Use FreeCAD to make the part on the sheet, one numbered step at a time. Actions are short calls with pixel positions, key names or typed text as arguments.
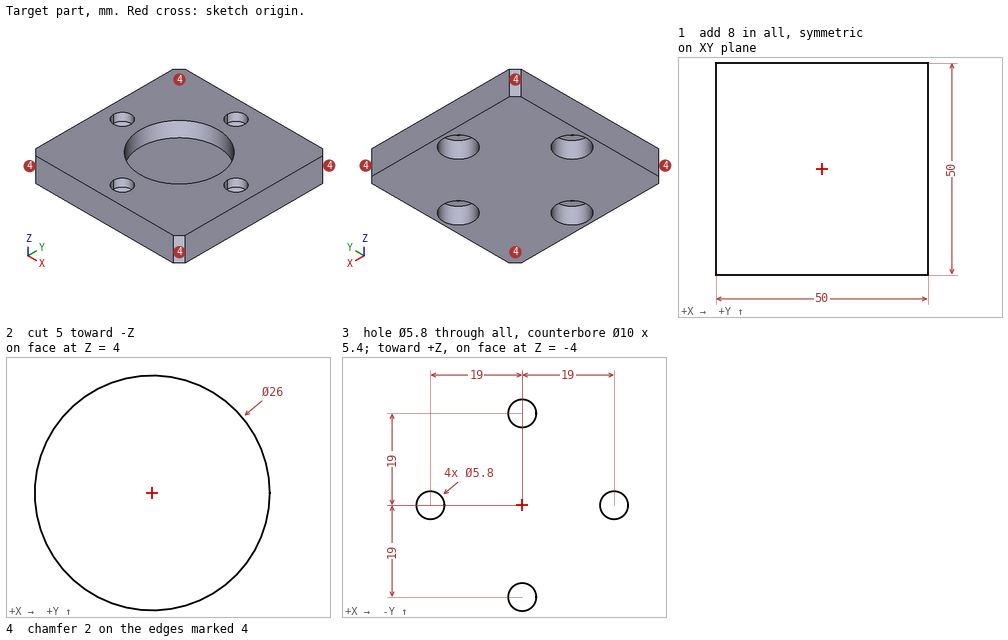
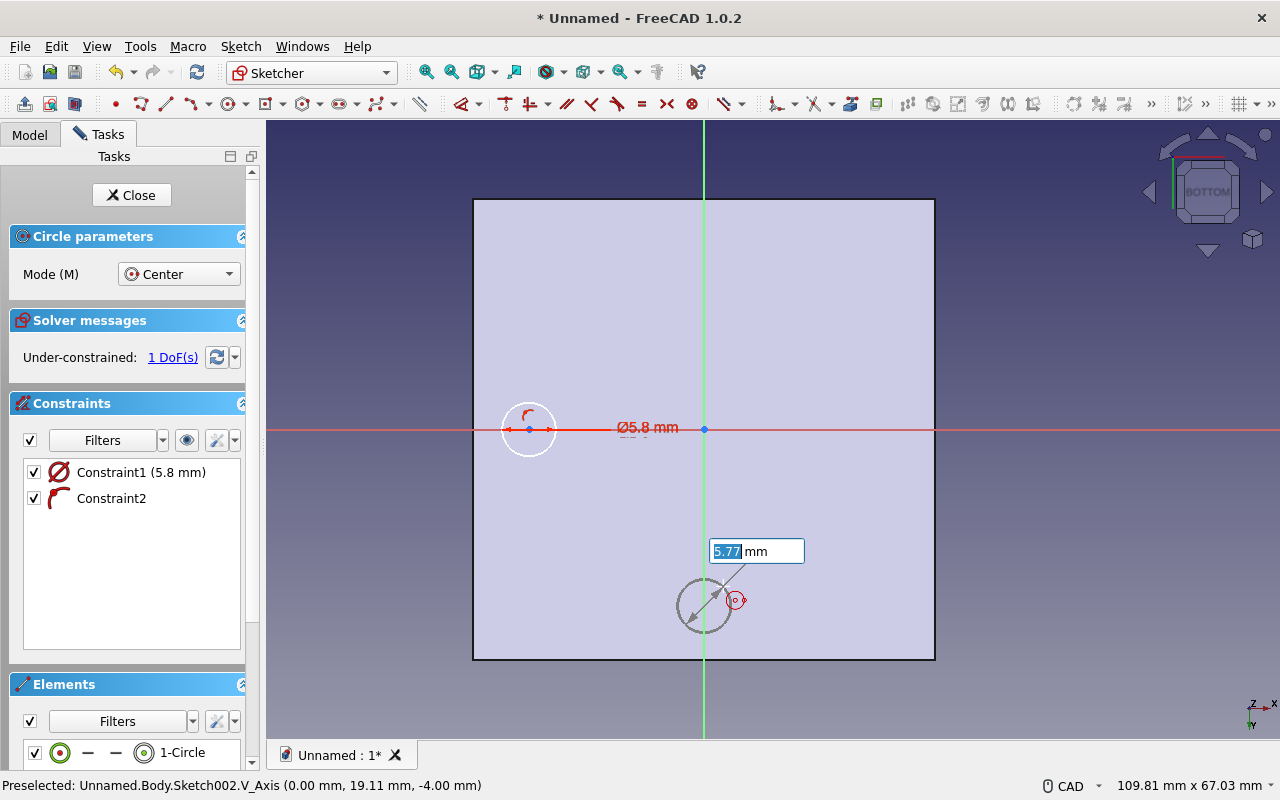
text(5.8)
key(Return)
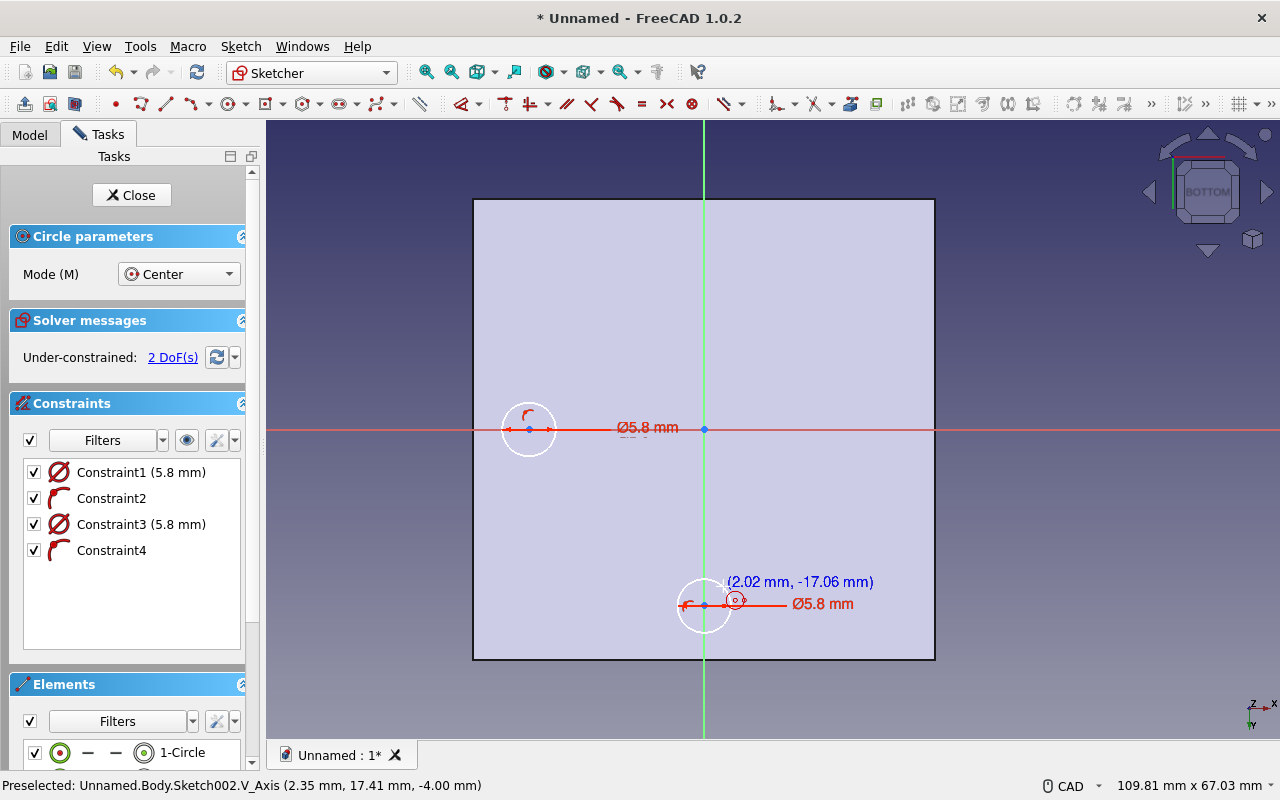
click(880, 430)
move(899, 411)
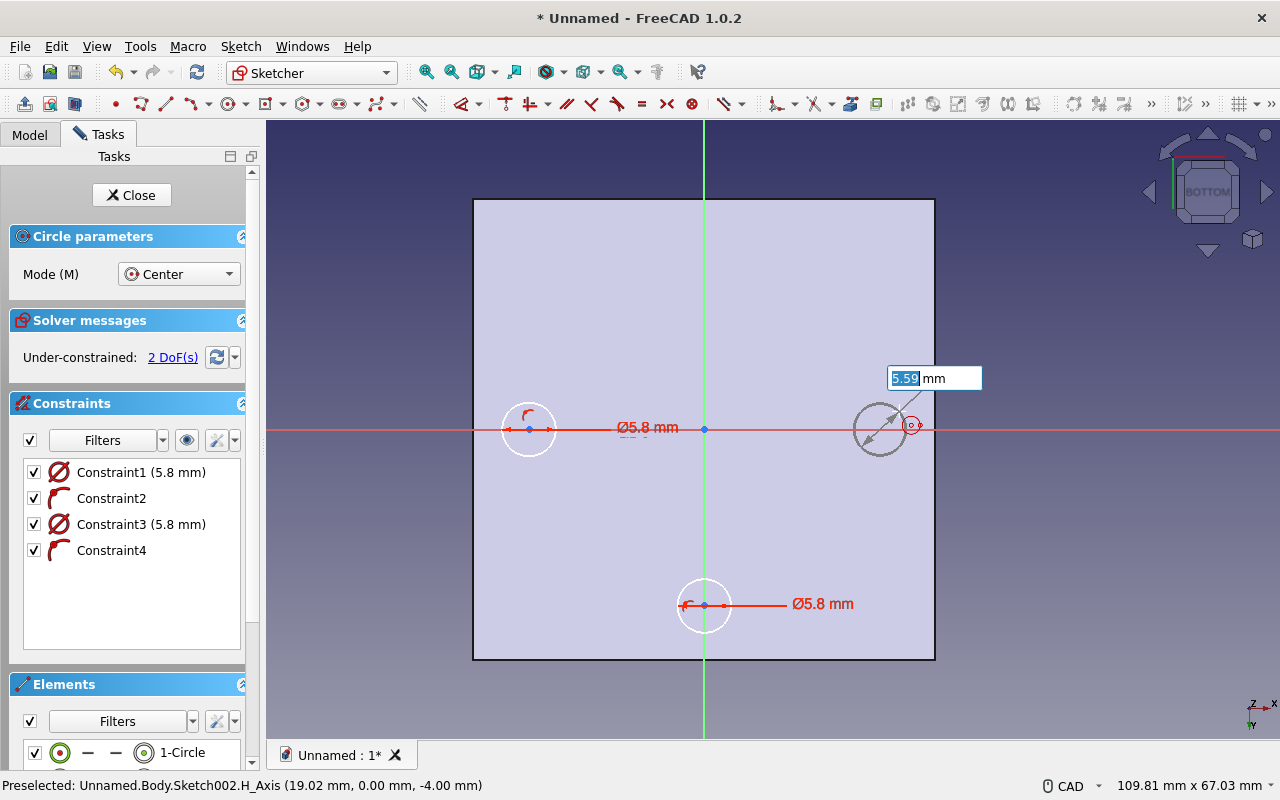
text(5.8)
key(Return)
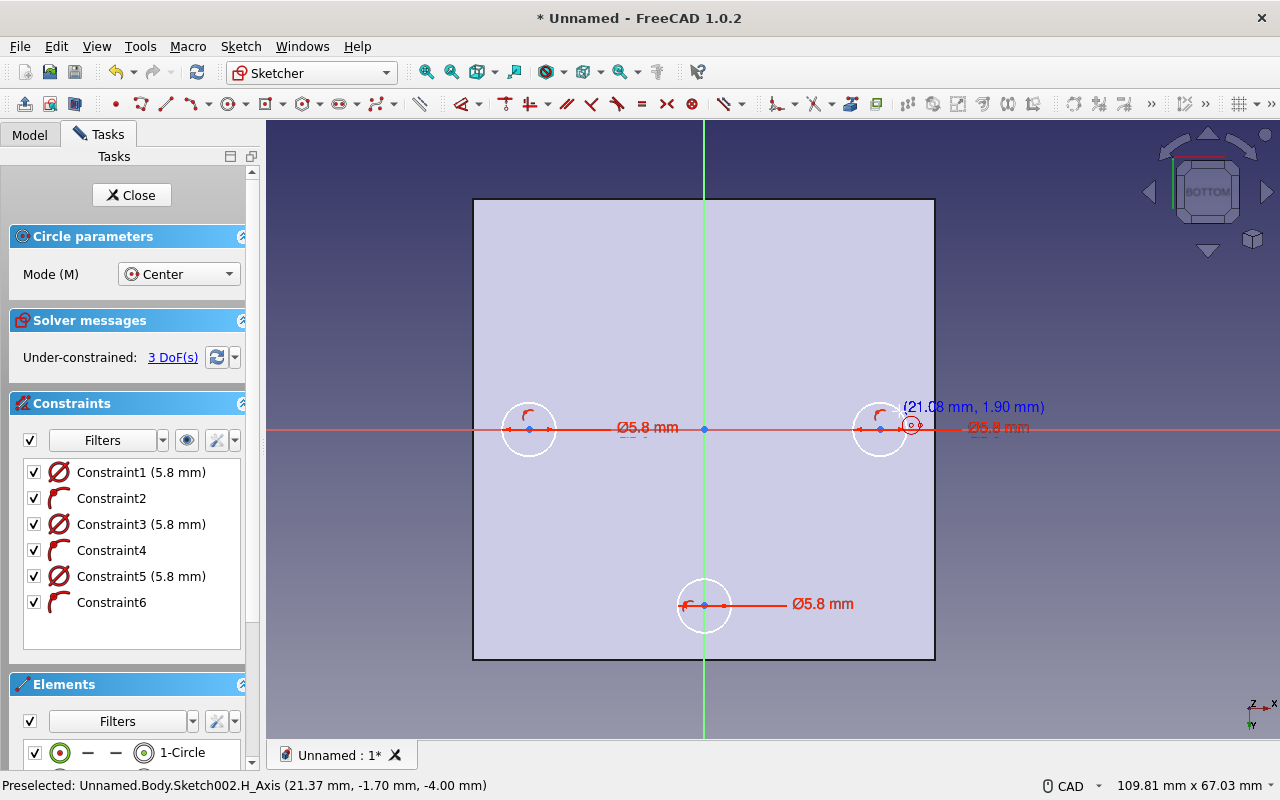
click(704, 254)
move(723, 235)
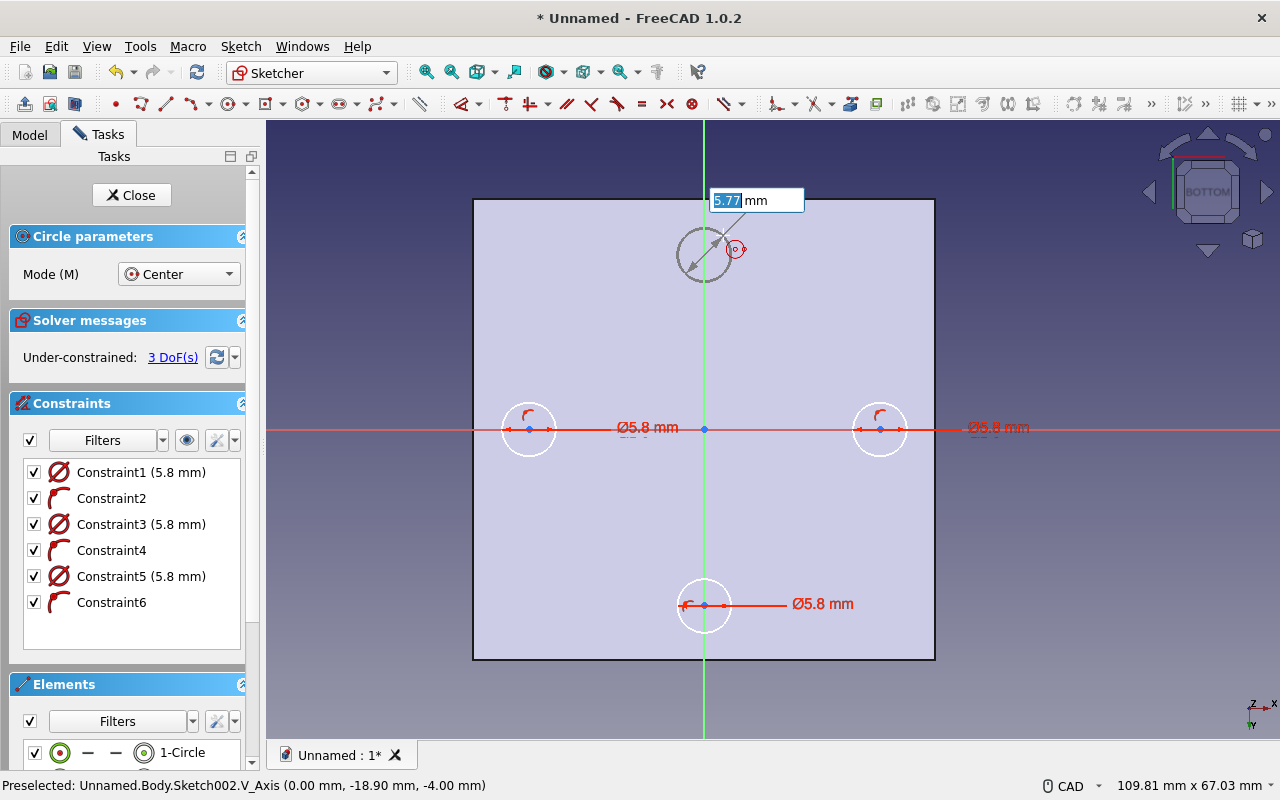
text(5.8)
key(Return)
key(Escape)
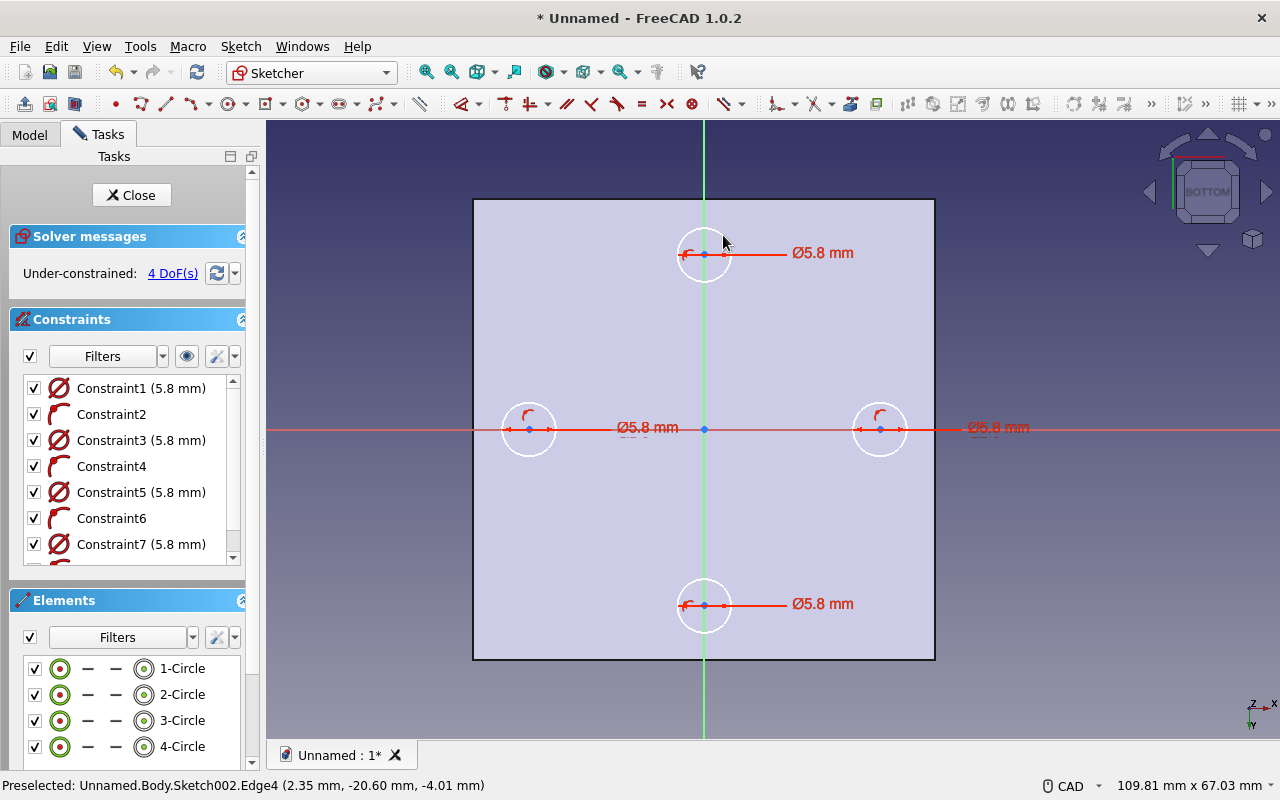
click(529, 430)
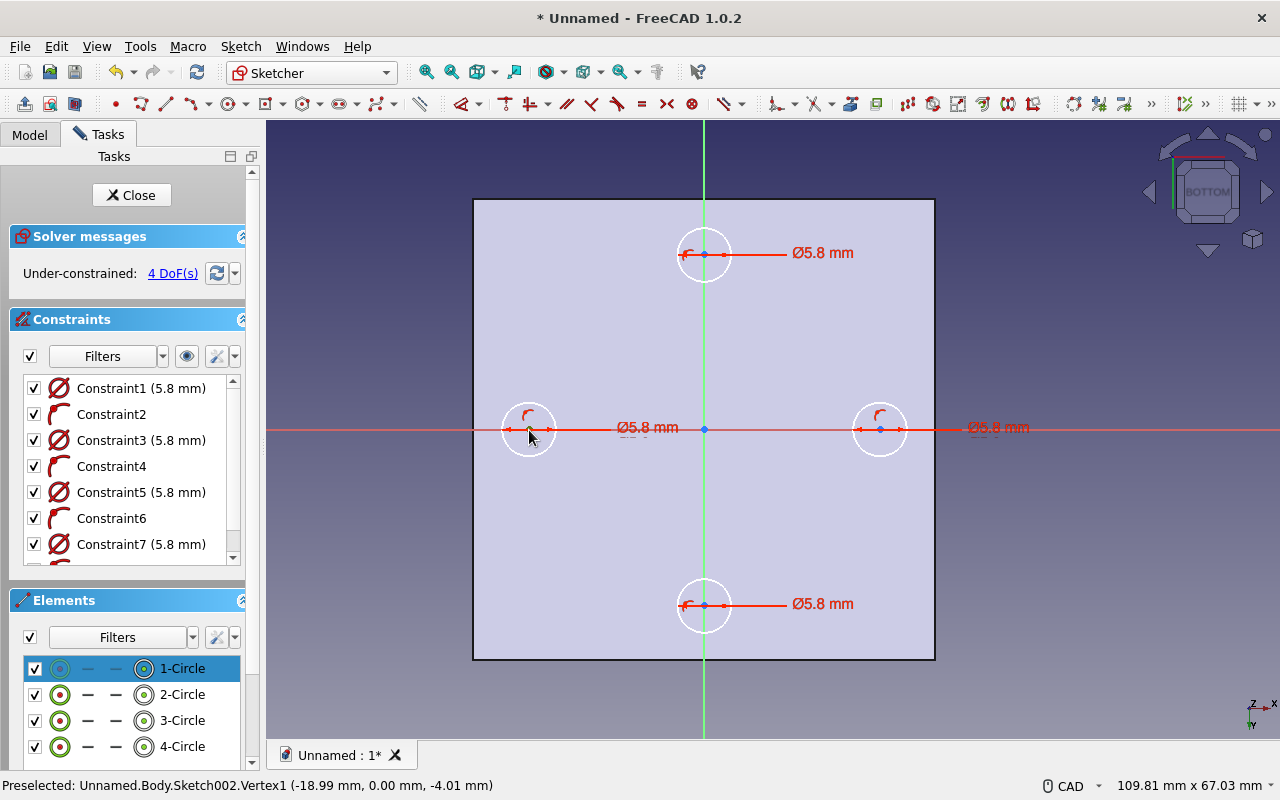
click(478, 104)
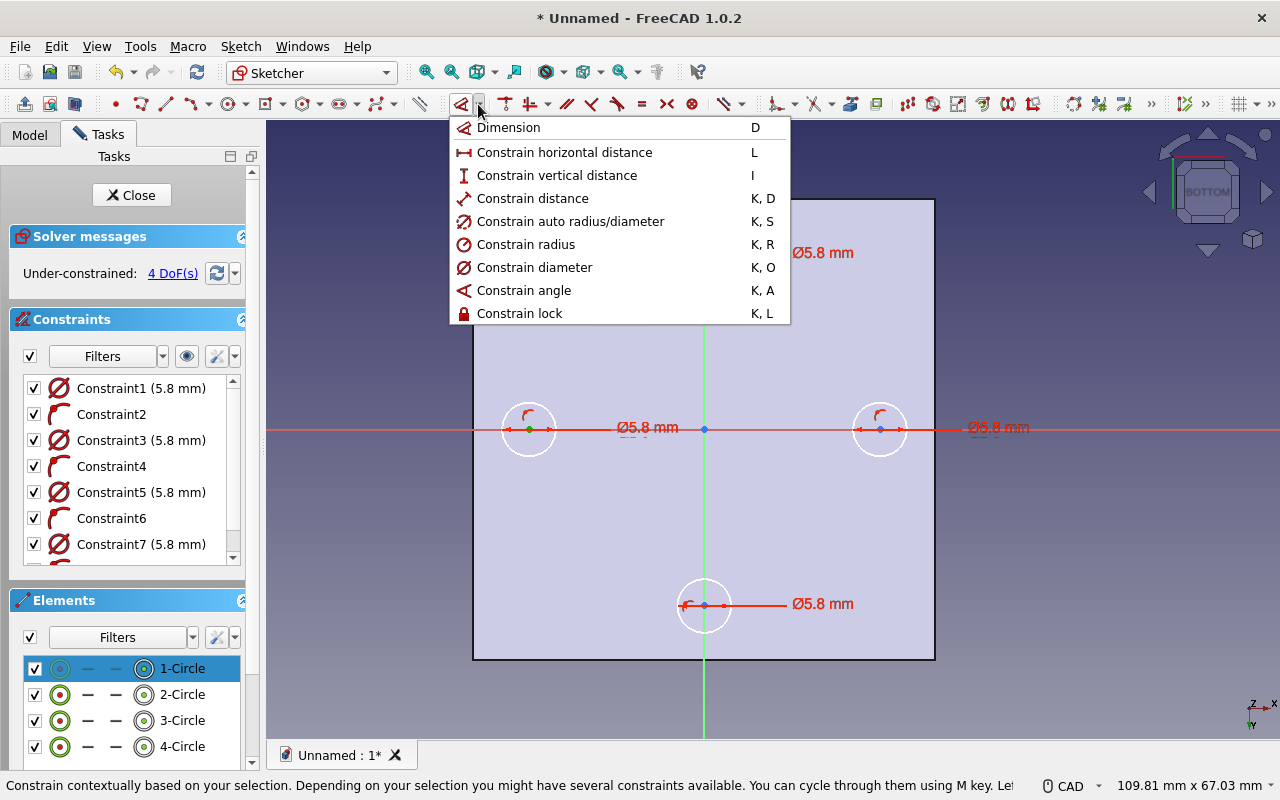
click(620, 152)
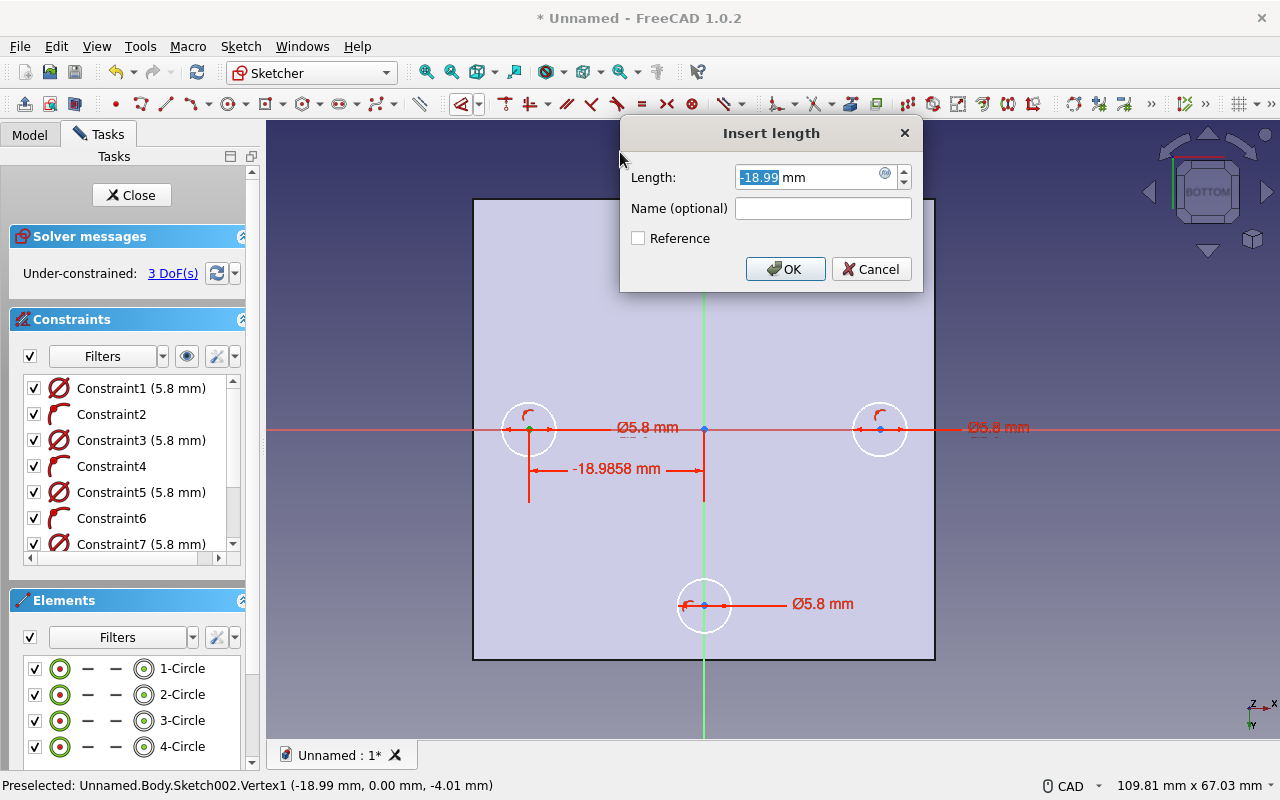
text(-19)
key(Return)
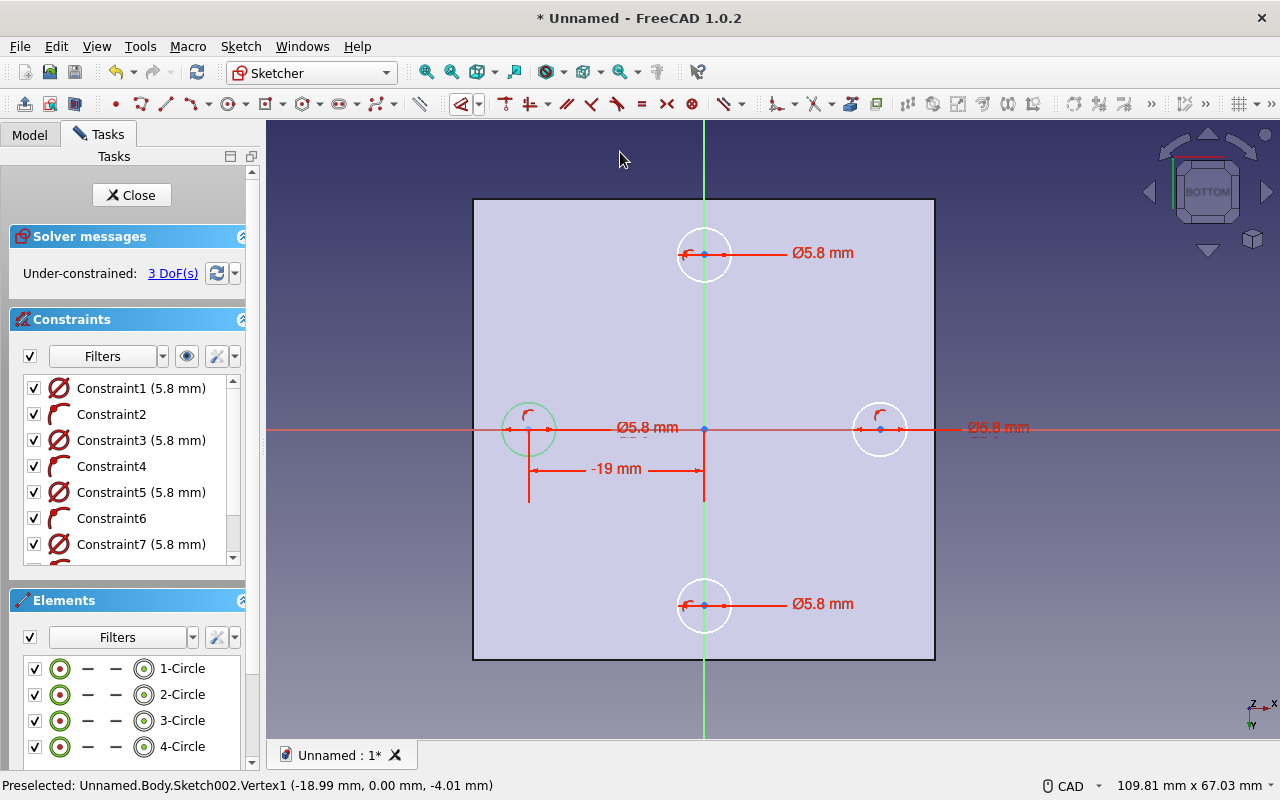
click(704, 606)